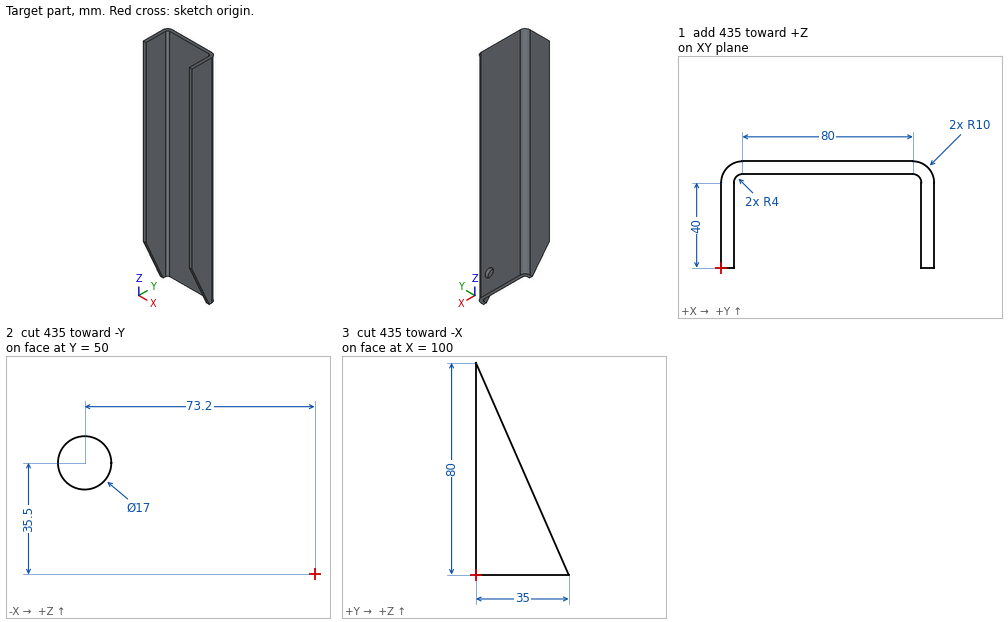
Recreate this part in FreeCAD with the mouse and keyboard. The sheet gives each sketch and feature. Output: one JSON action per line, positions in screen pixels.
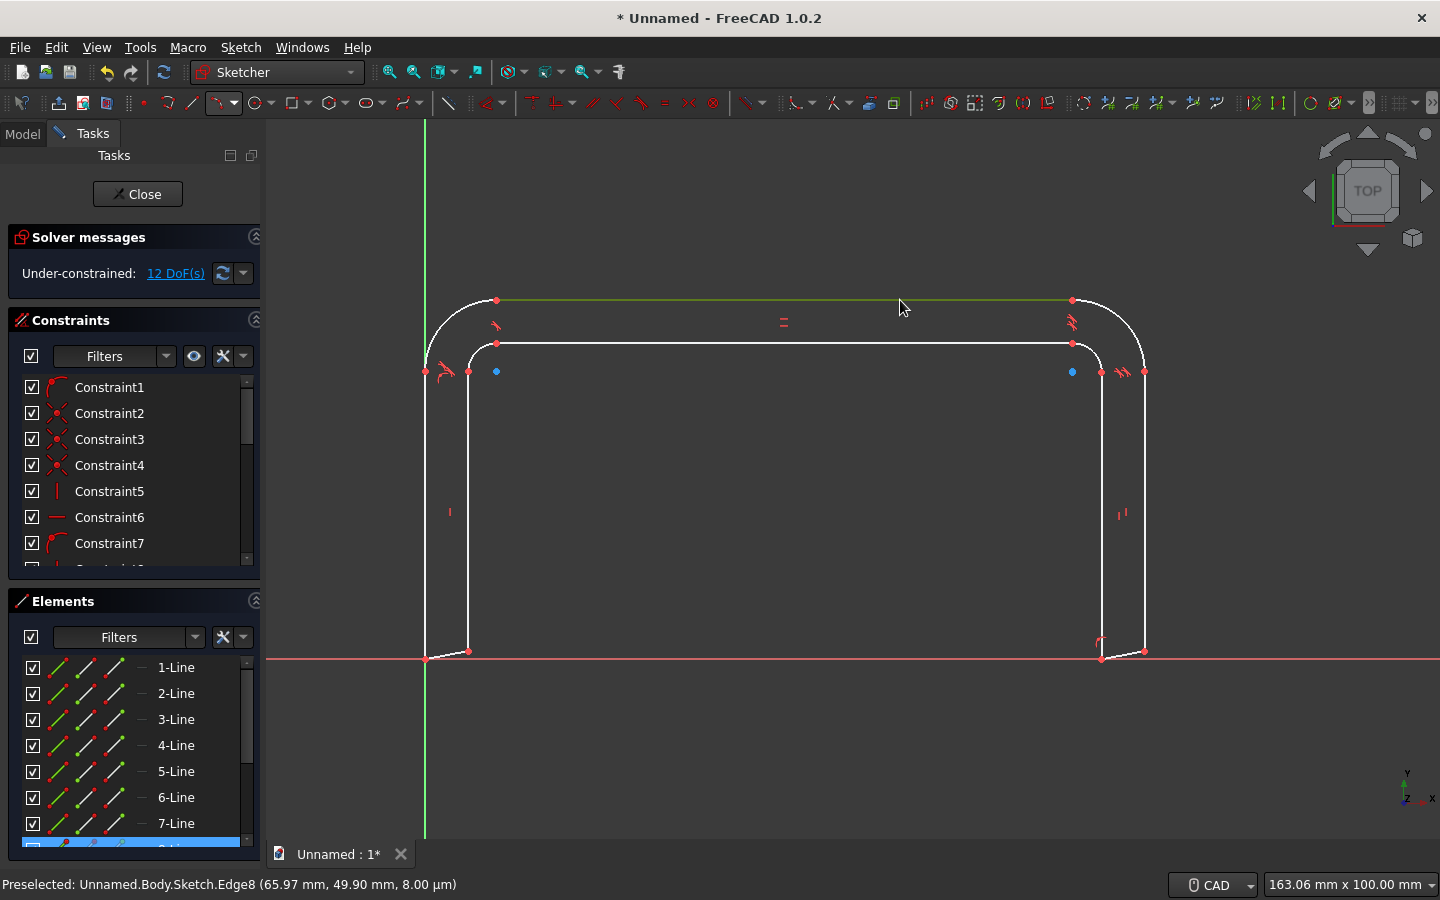
{"action": "left_click", "coordinate": [464, 308]}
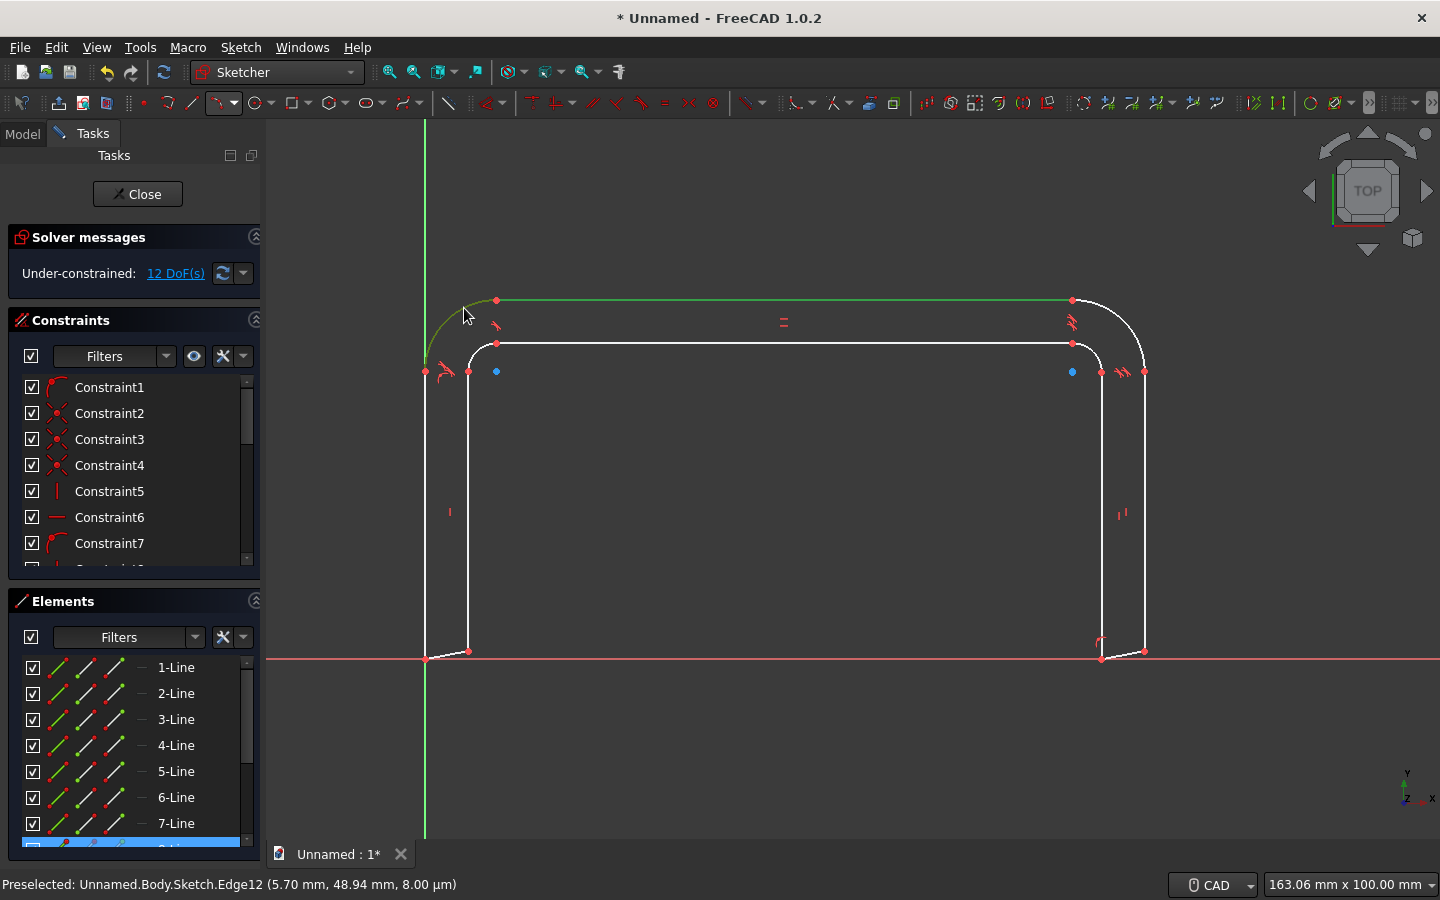
{"action": "left_click", "coordinate": [642, 104]}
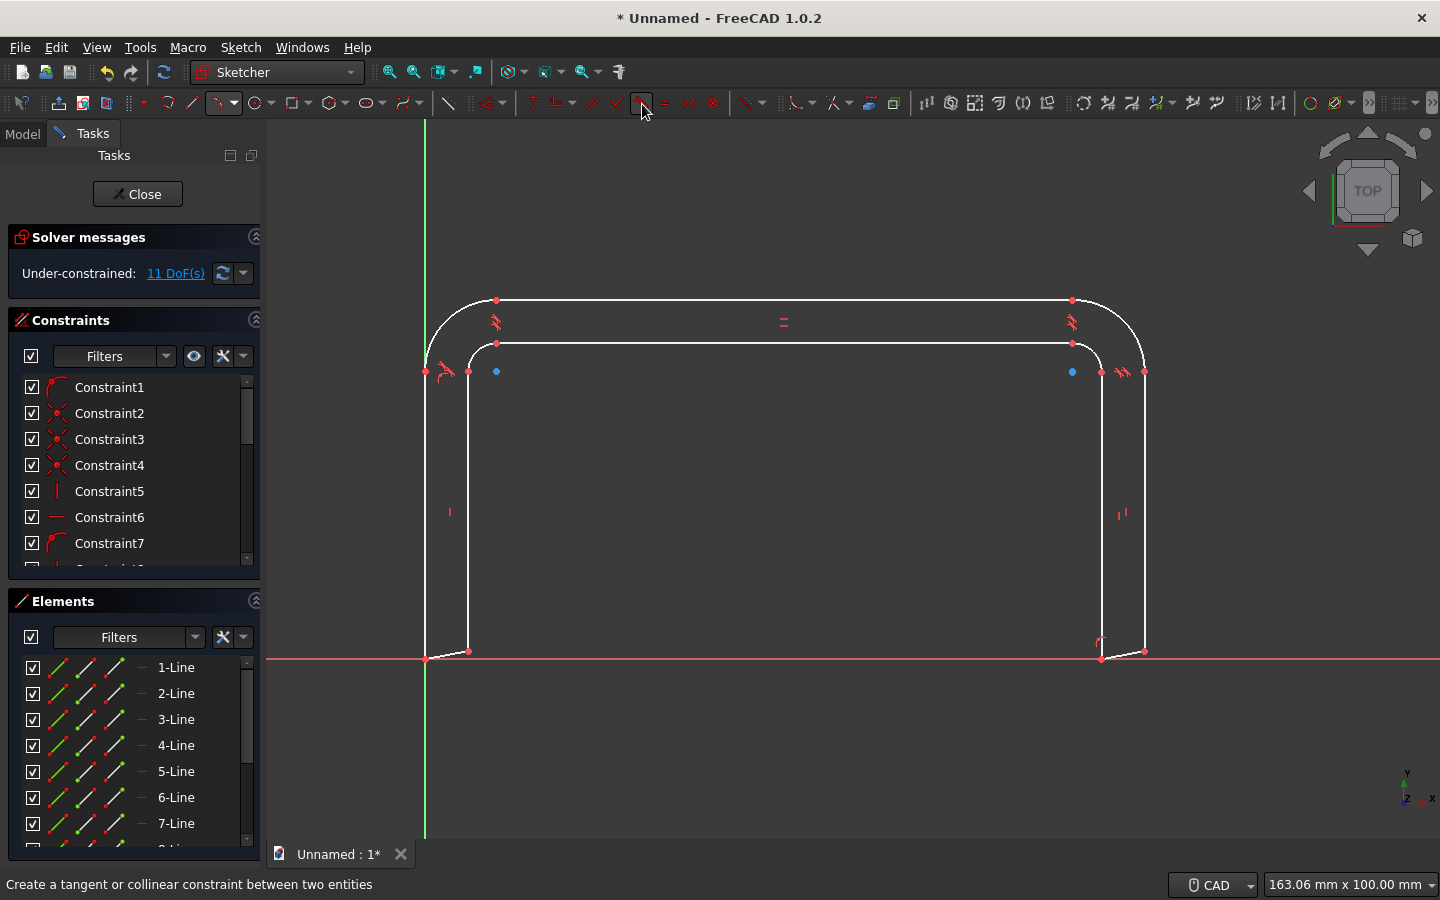
{"action": "left_click", "coordinate": [438, 657]}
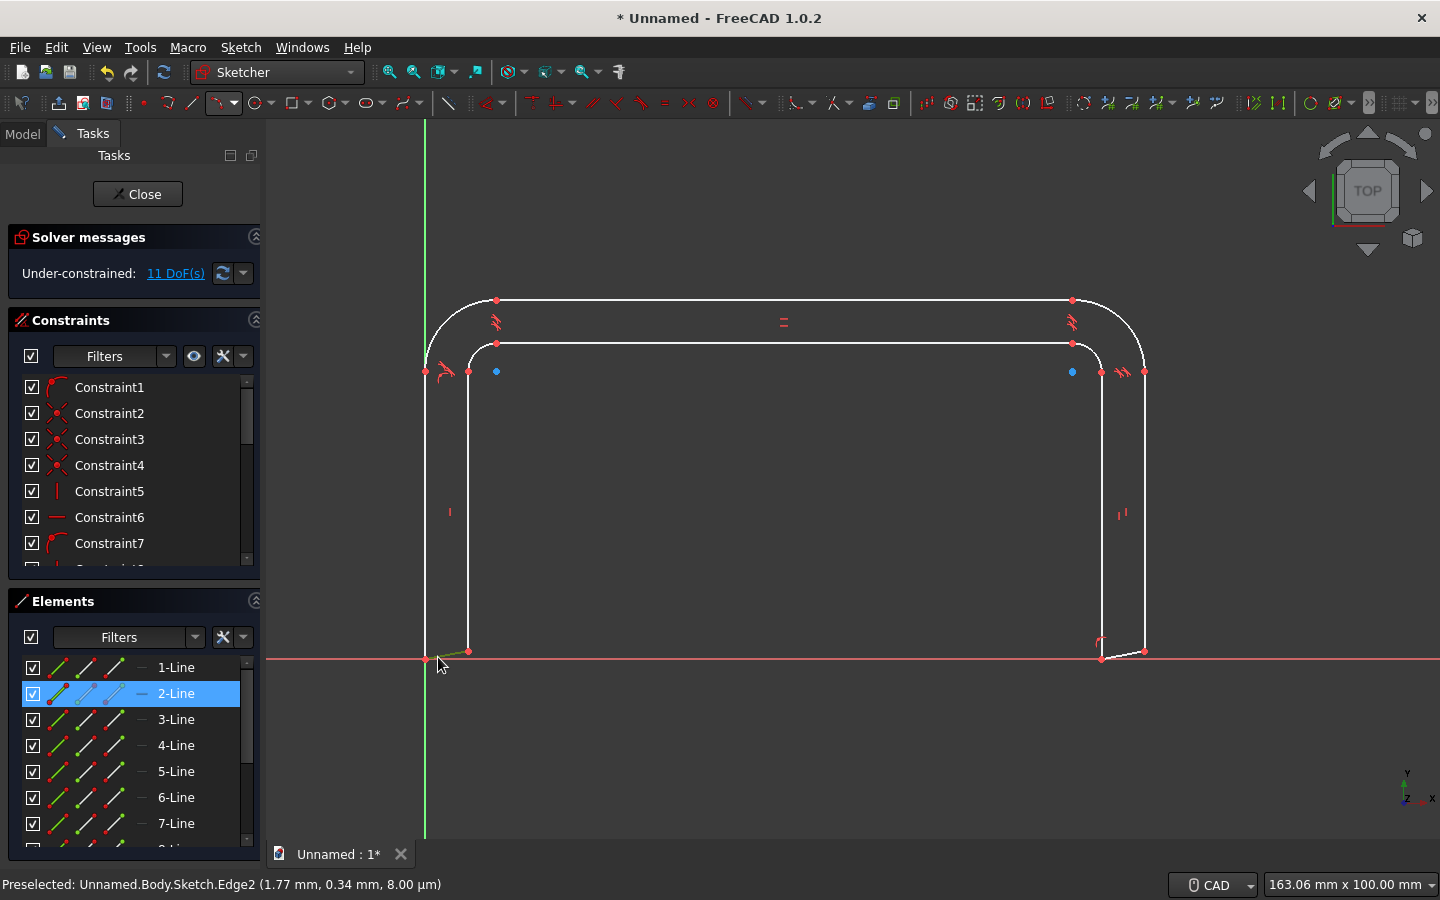
{"action": "left_click", "coordinate": [574, 104]}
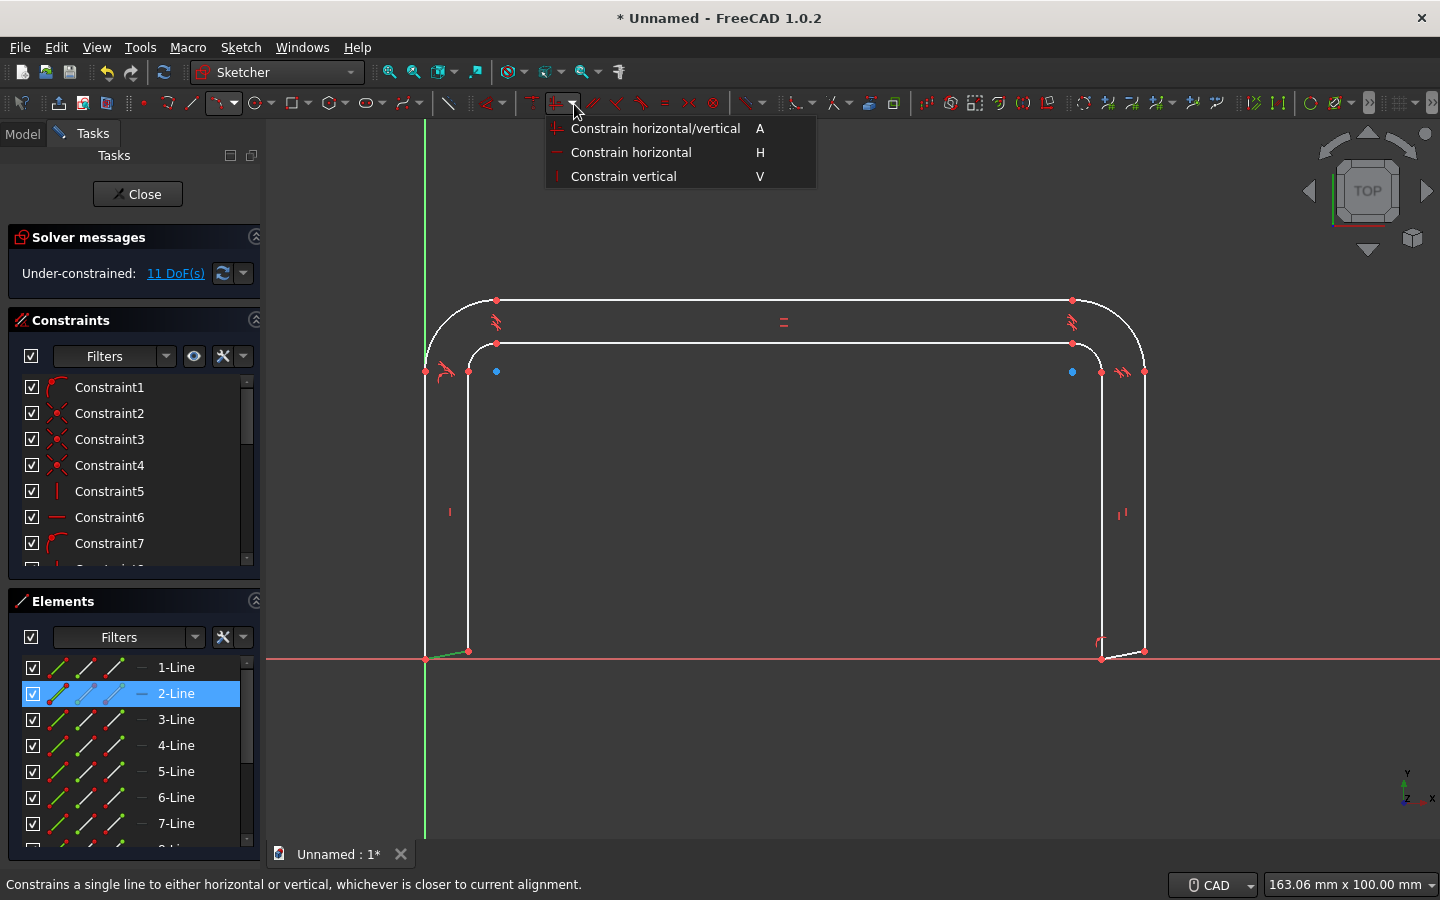
{"action": "left_click", "coordinate": [681, 152]}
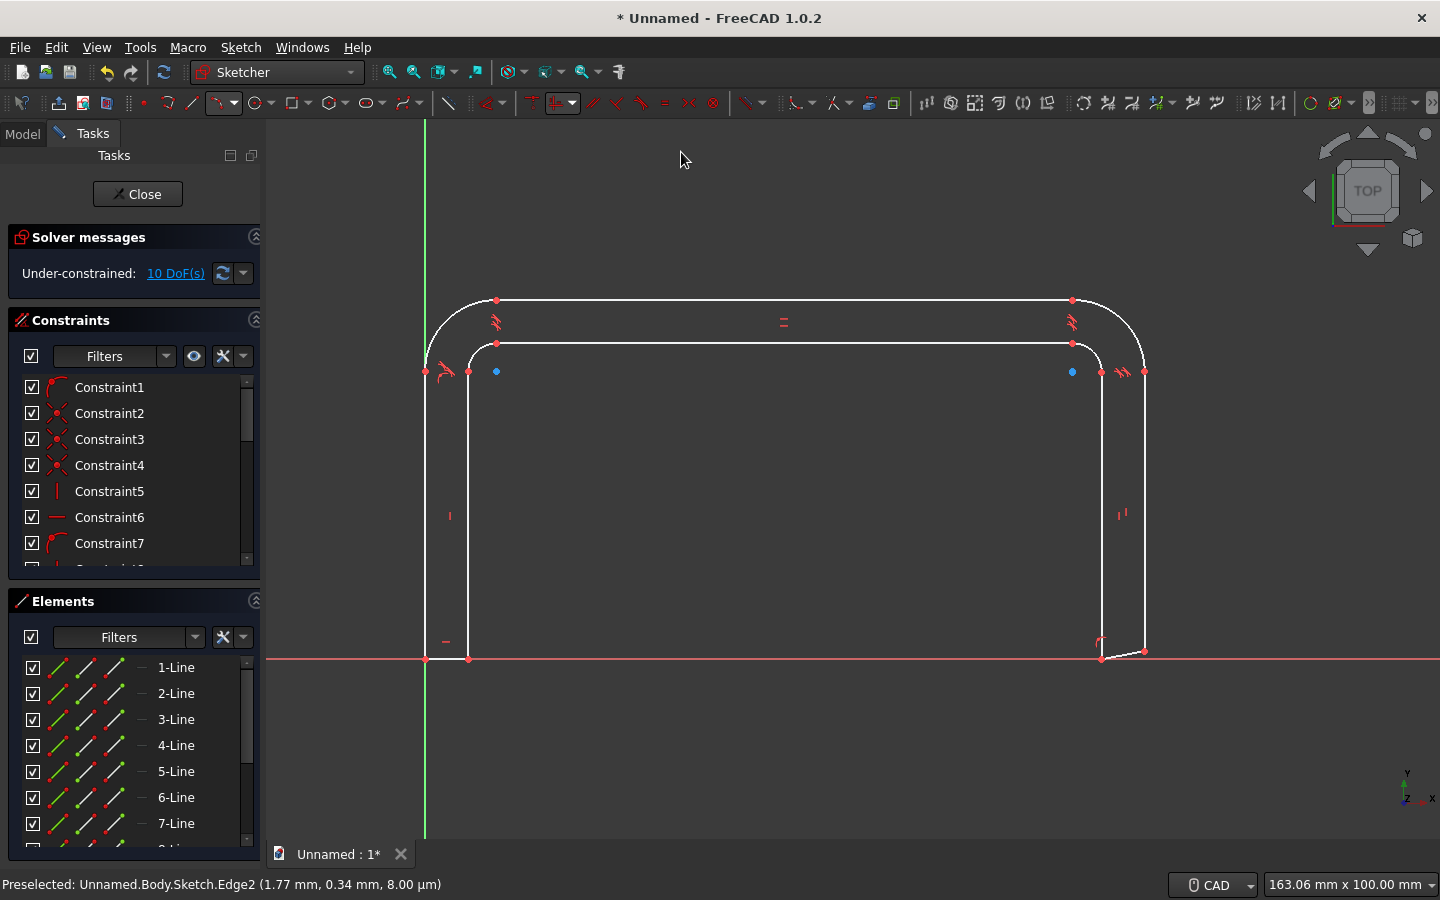
{"action": "left_click", "coordinate": [1115, 657]}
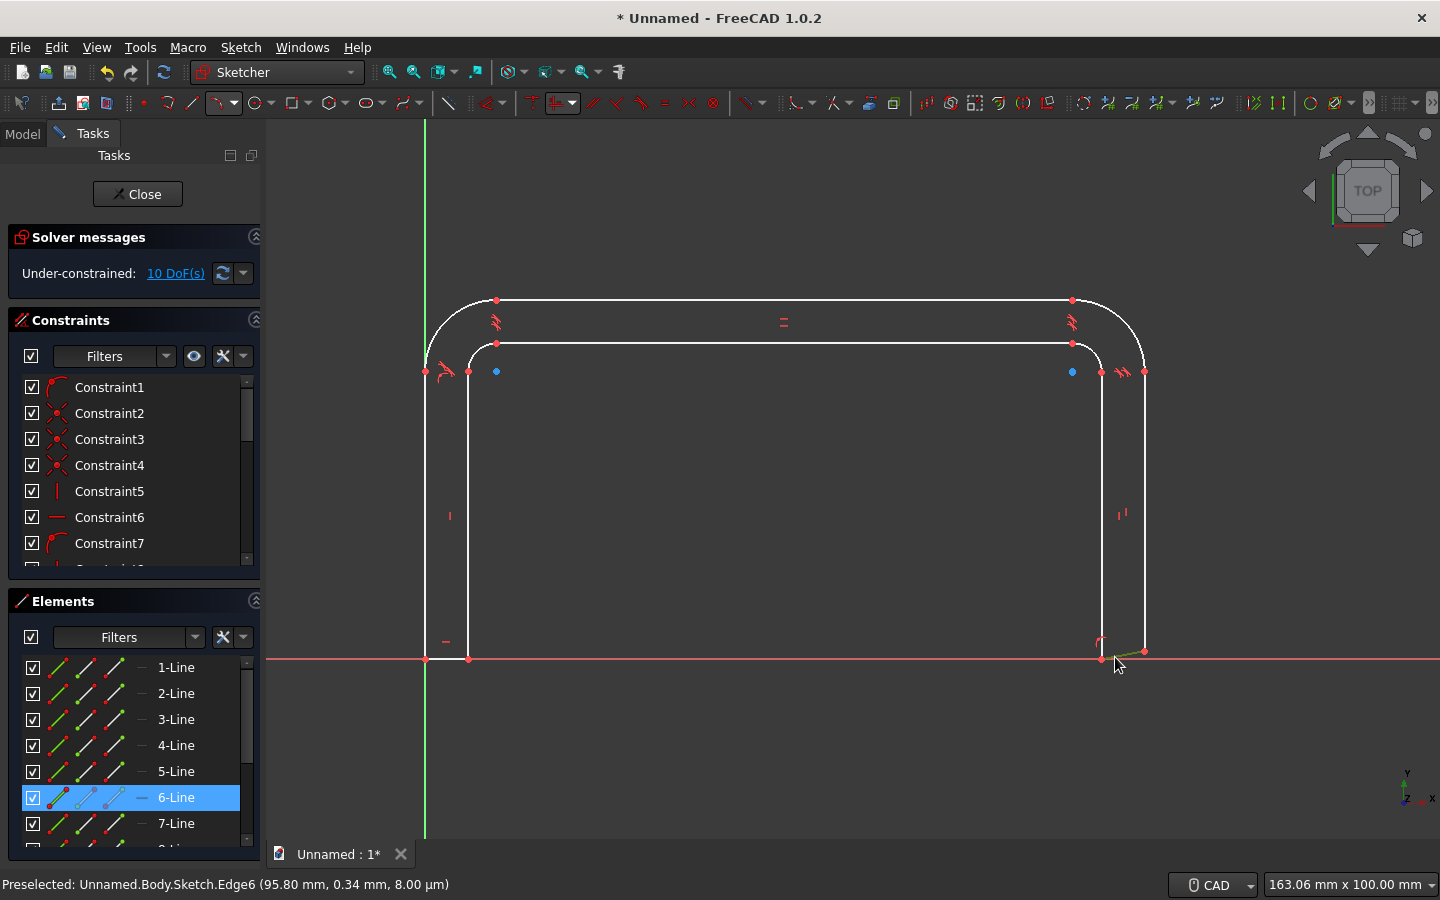
{"action": "key", "text": "h"}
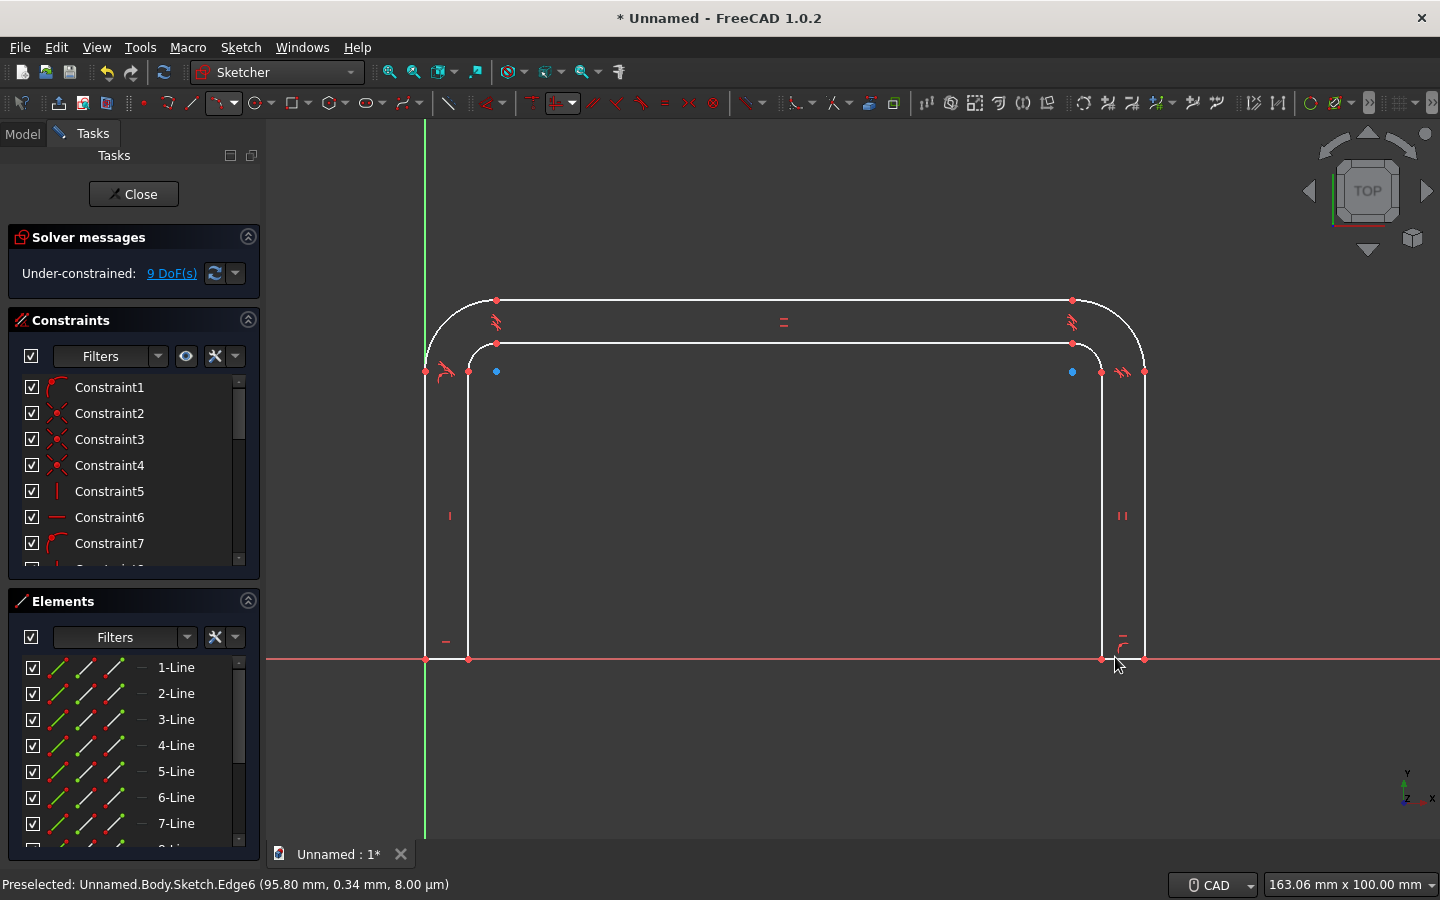
{"action": "left_click", "coordinate": [1099, 359]}